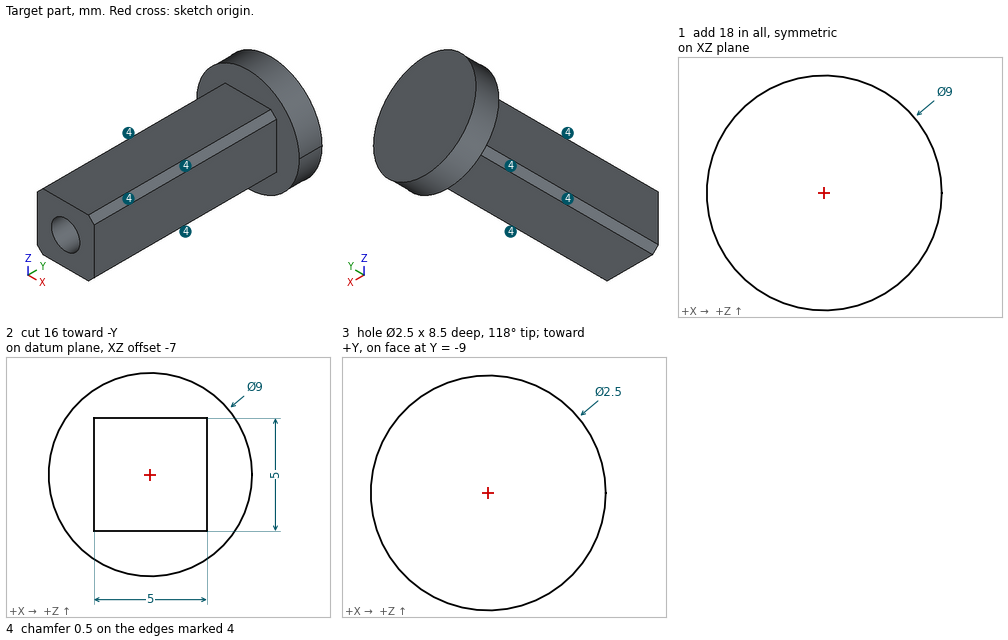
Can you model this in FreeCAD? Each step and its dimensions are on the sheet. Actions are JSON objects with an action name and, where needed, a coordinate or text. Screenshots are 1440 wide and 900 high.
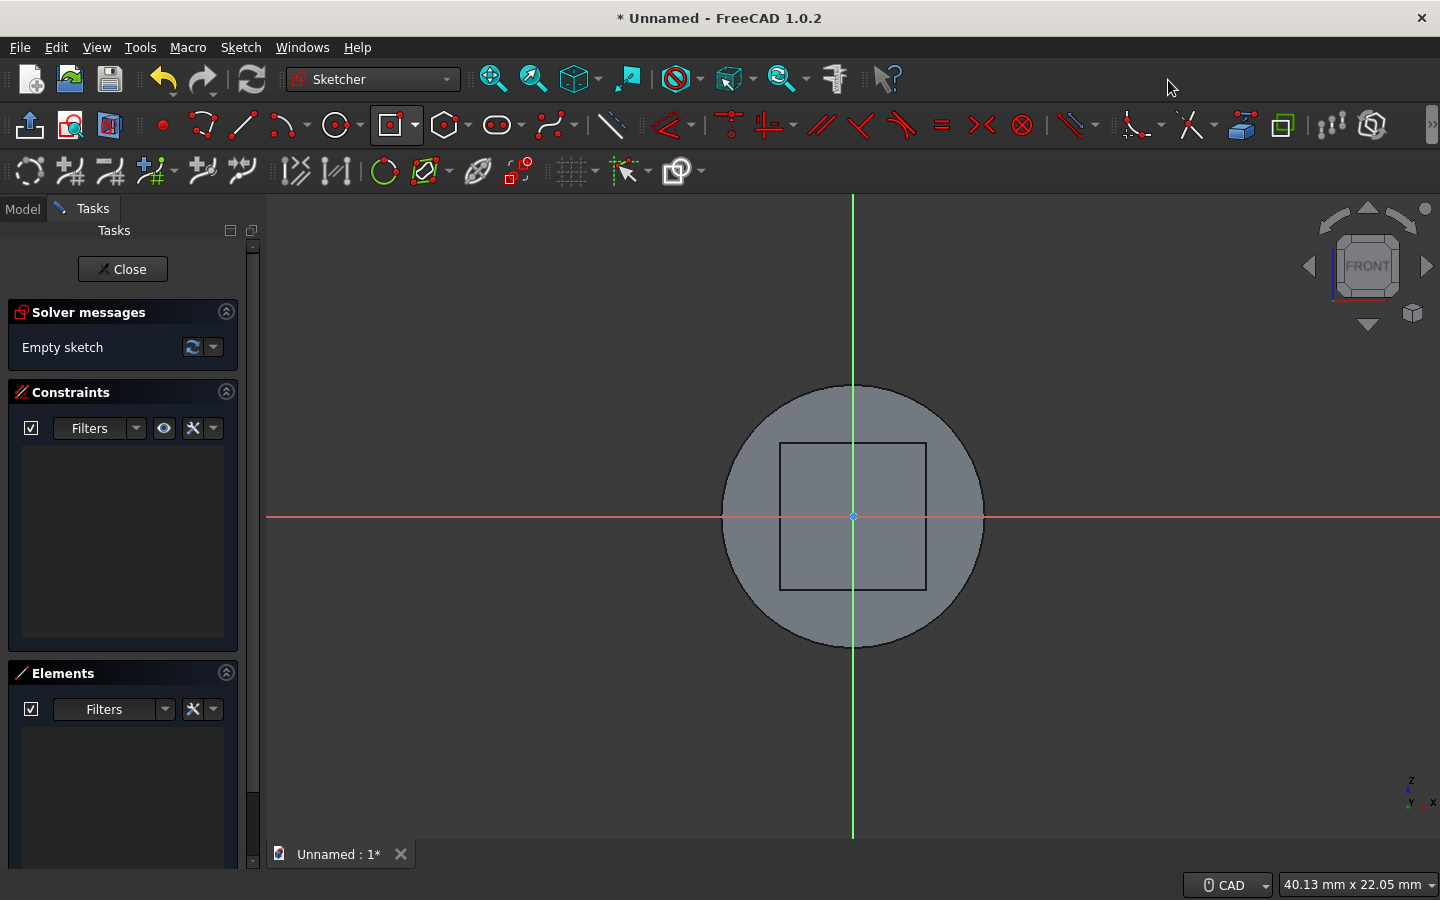
{"action": "scroll", "coordinate": [867, 516], "scroll_direction": "up", "scroll_amount": 9}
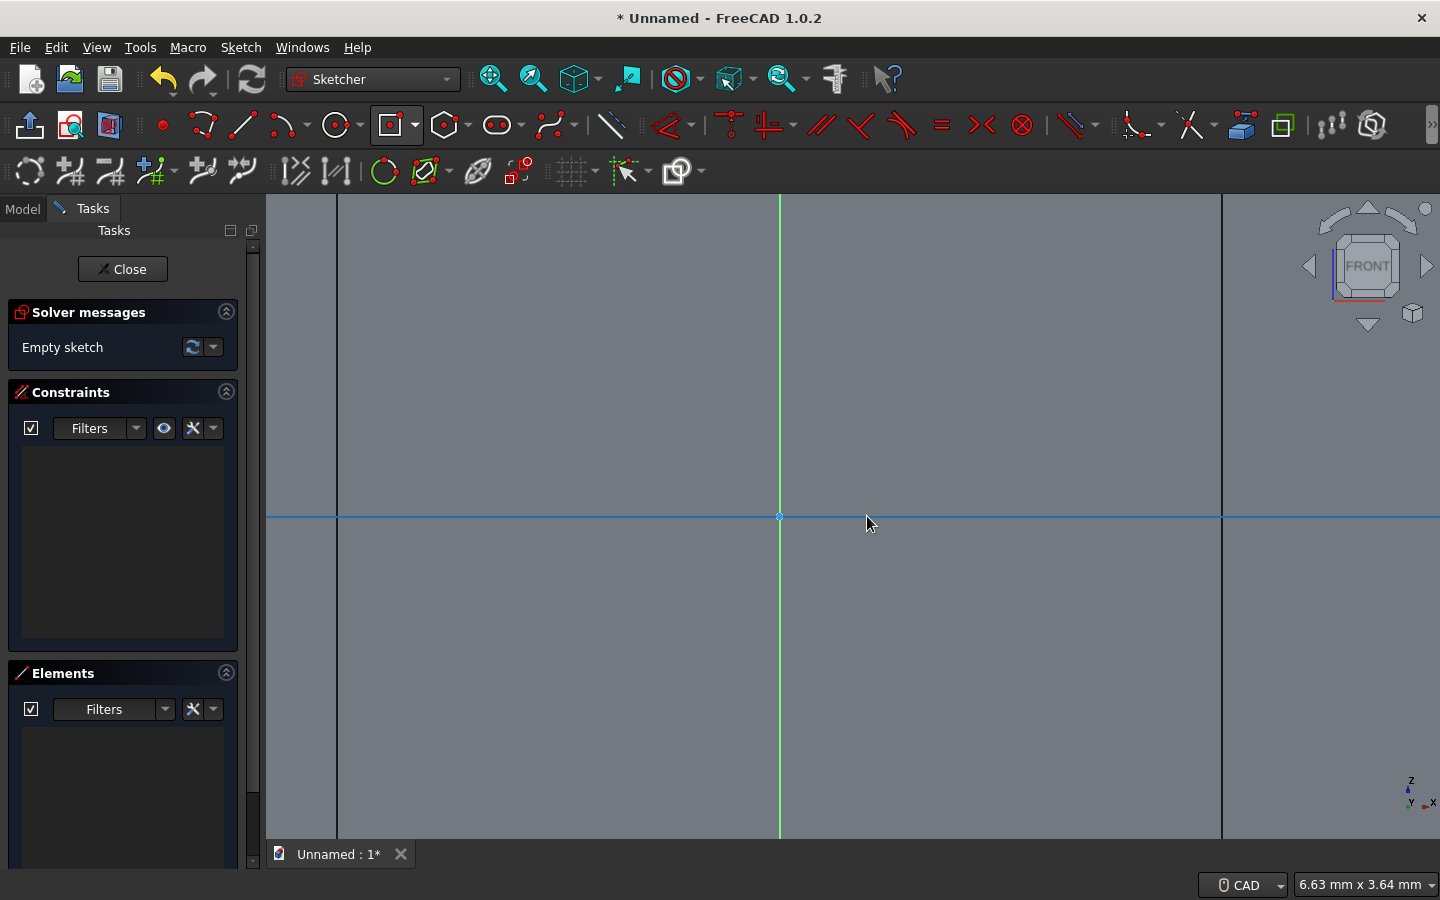
{"action": "left_click", "coordinate": [336, 126]}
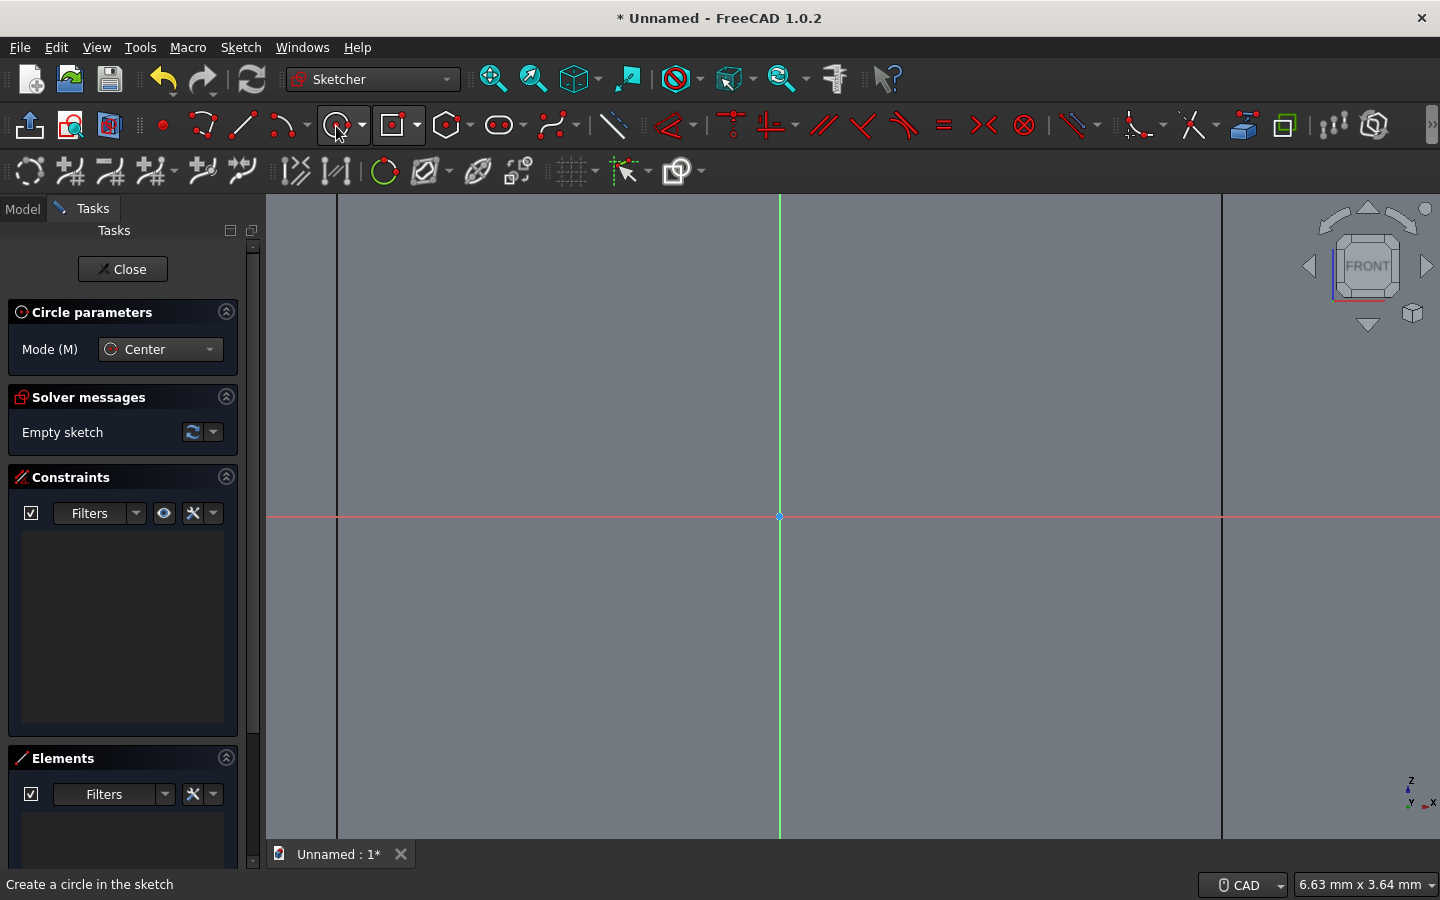
{"action": "left_click", "coordinate": [780, 516]}
{"action": "mouse_move", "coordinate": [936, 360]}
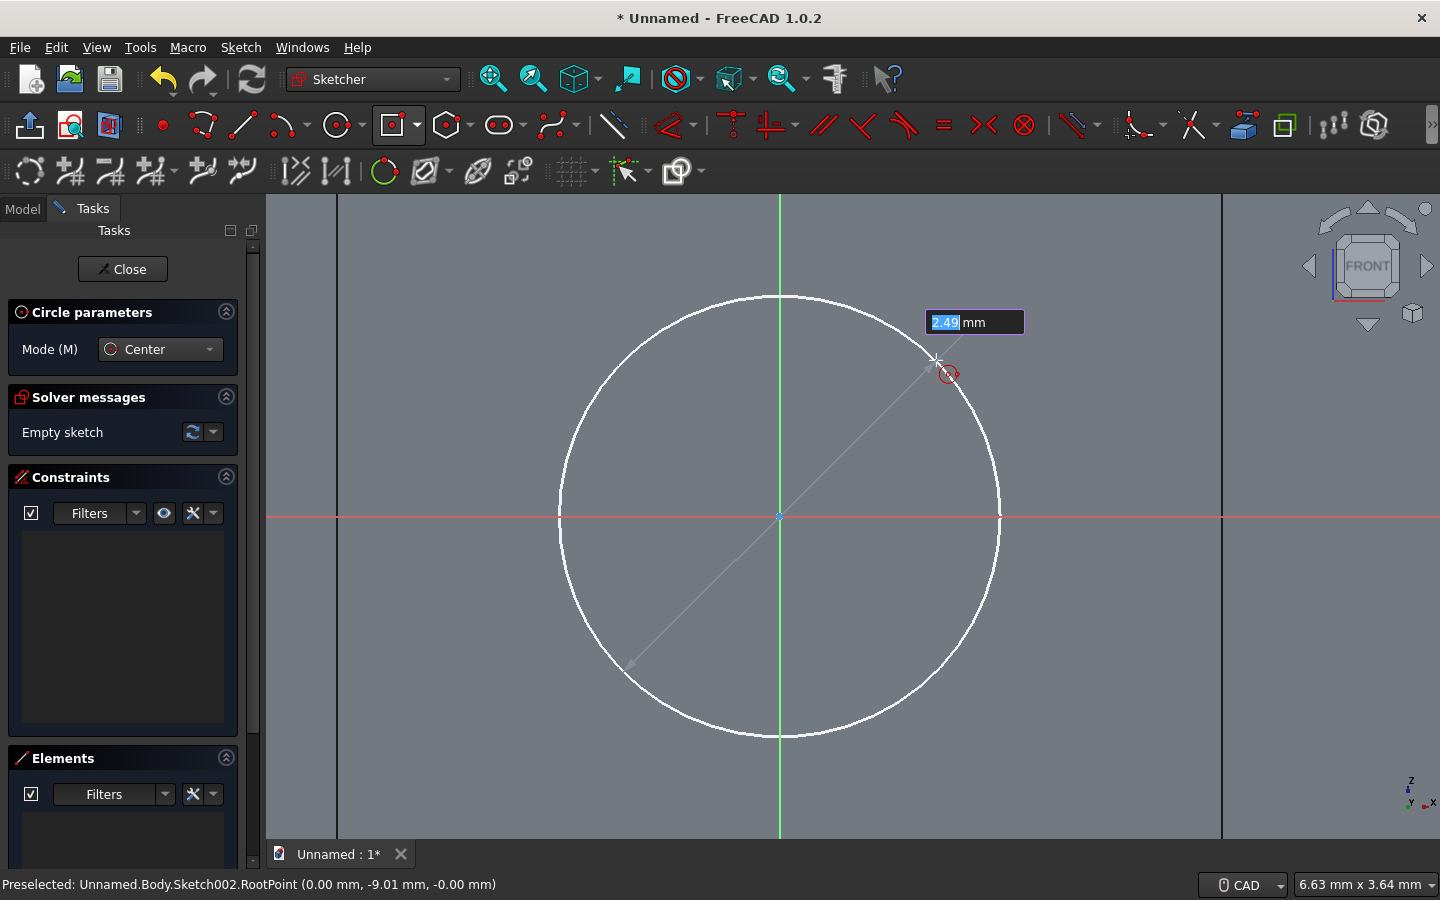
{"action": "type", "text": "2.5"}
{"action": "key", "text": "Return"}
{"action": "key", "text": "Escape"}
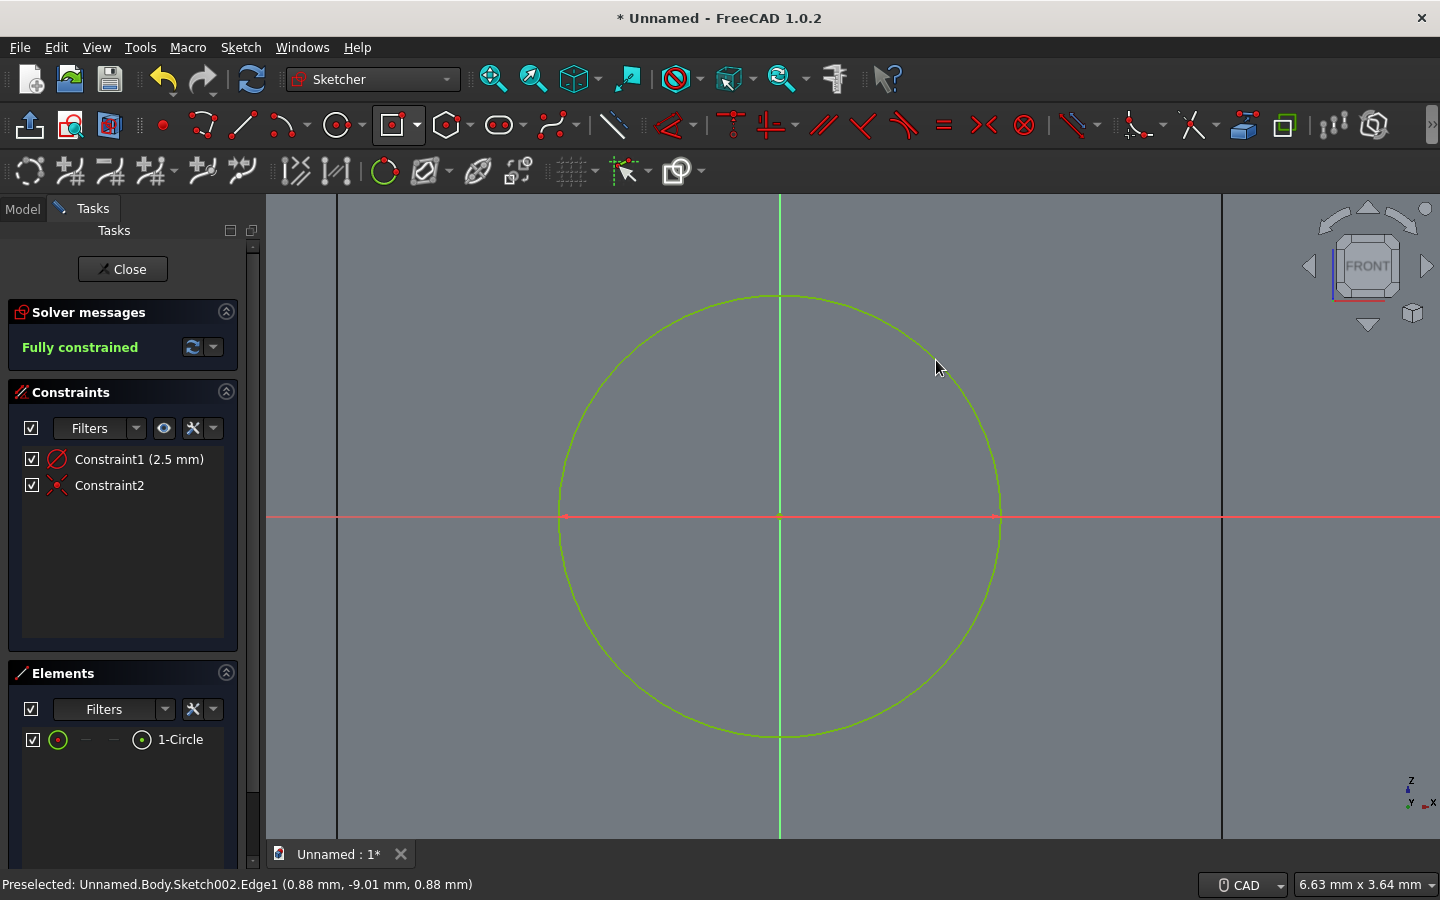
{"action": "left_click", "coordinate": [123, 269]}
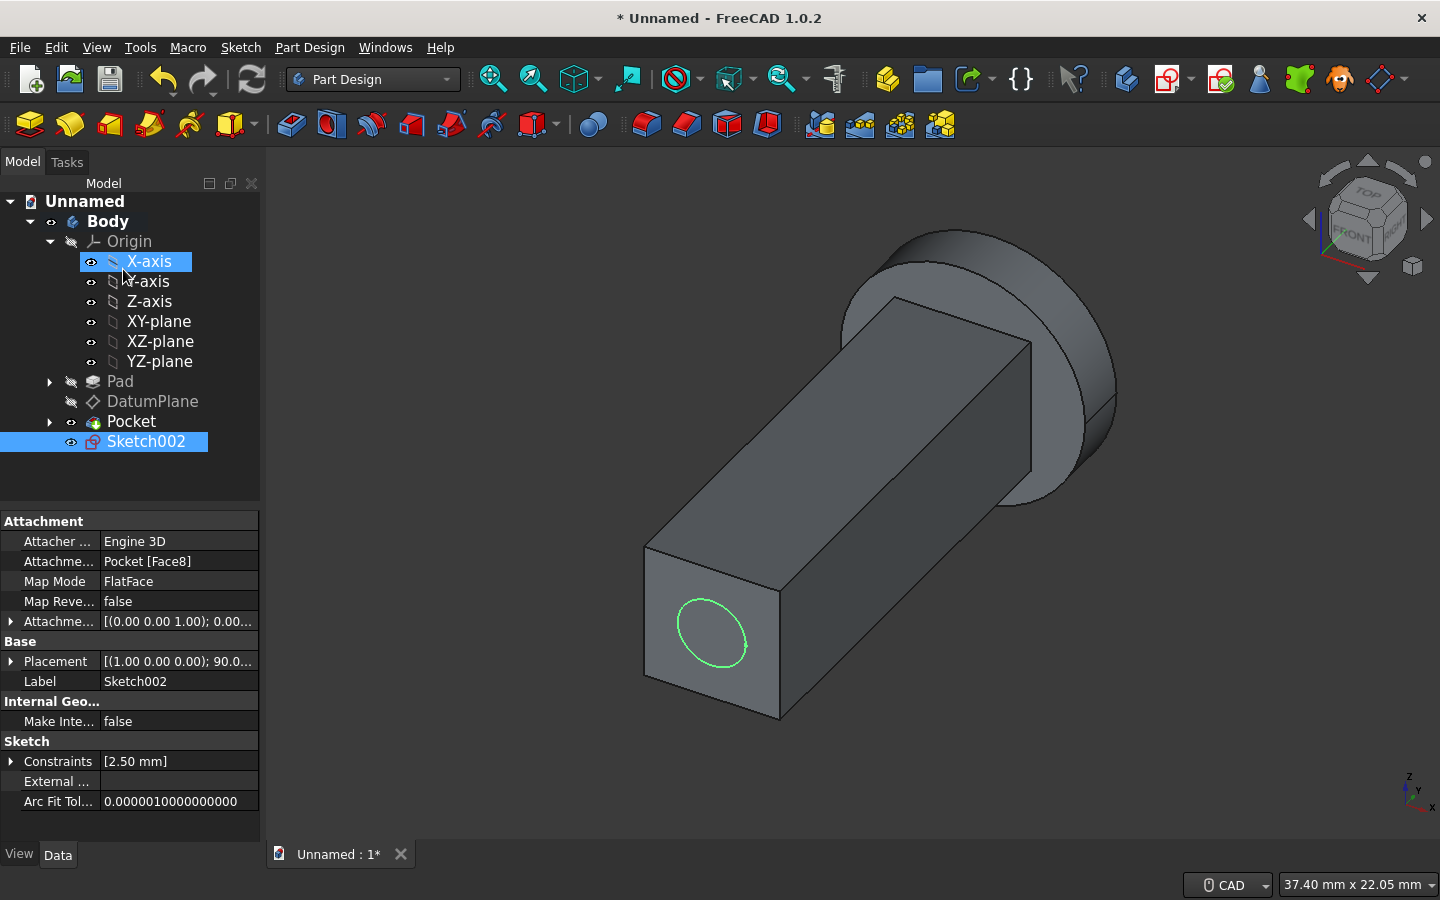
{"action": "left_click", "coordinate": [332, 124]}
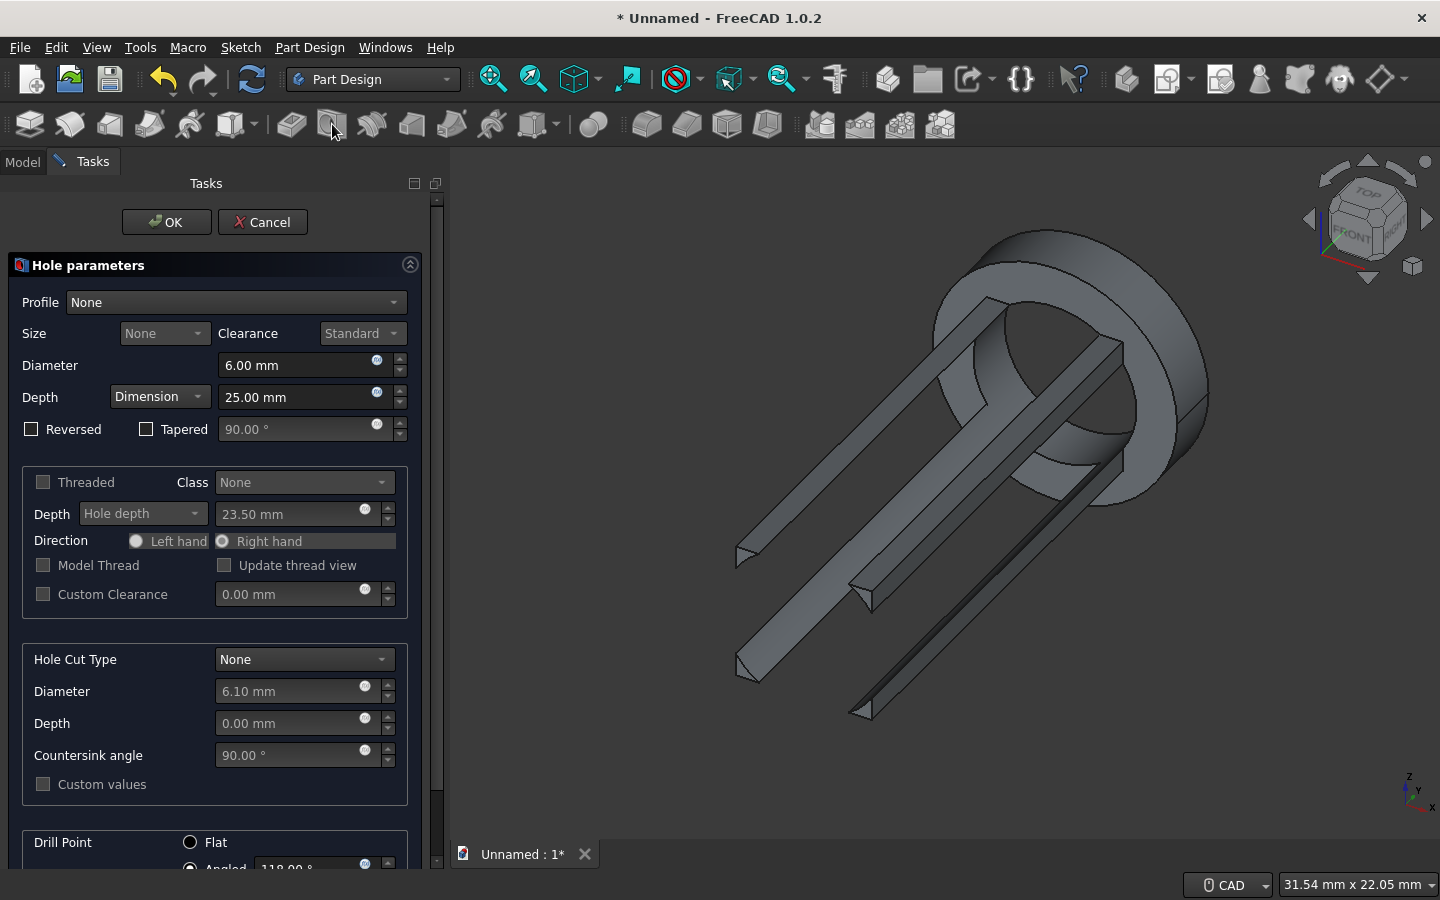
{"action": "triple_click", "coordinate": [305, 365]}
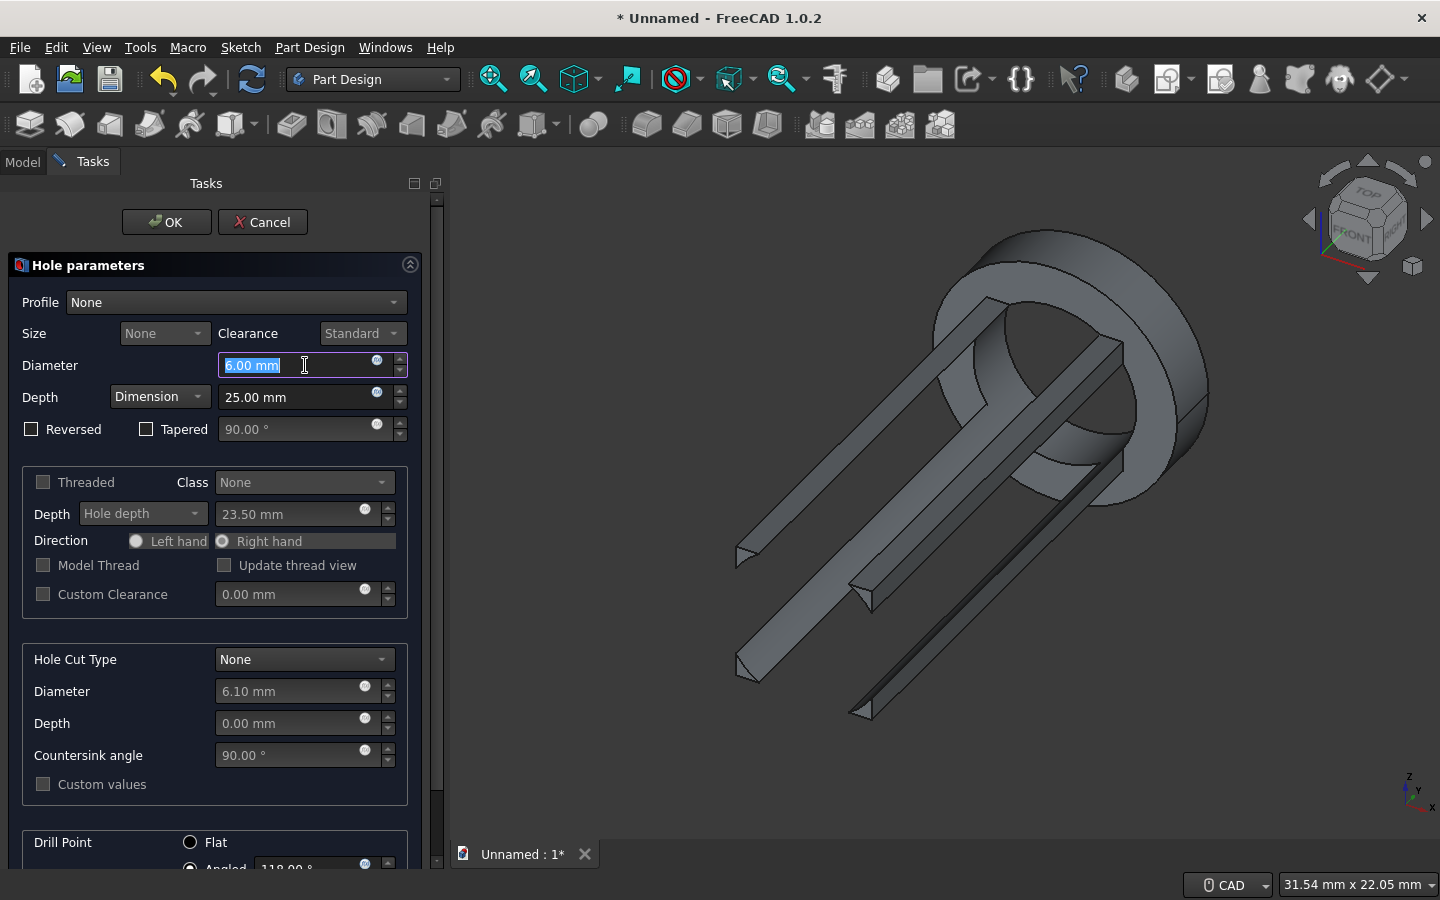
{"action": "type", "text": "2.5"}
{"action": "key", "text": "Tab"}